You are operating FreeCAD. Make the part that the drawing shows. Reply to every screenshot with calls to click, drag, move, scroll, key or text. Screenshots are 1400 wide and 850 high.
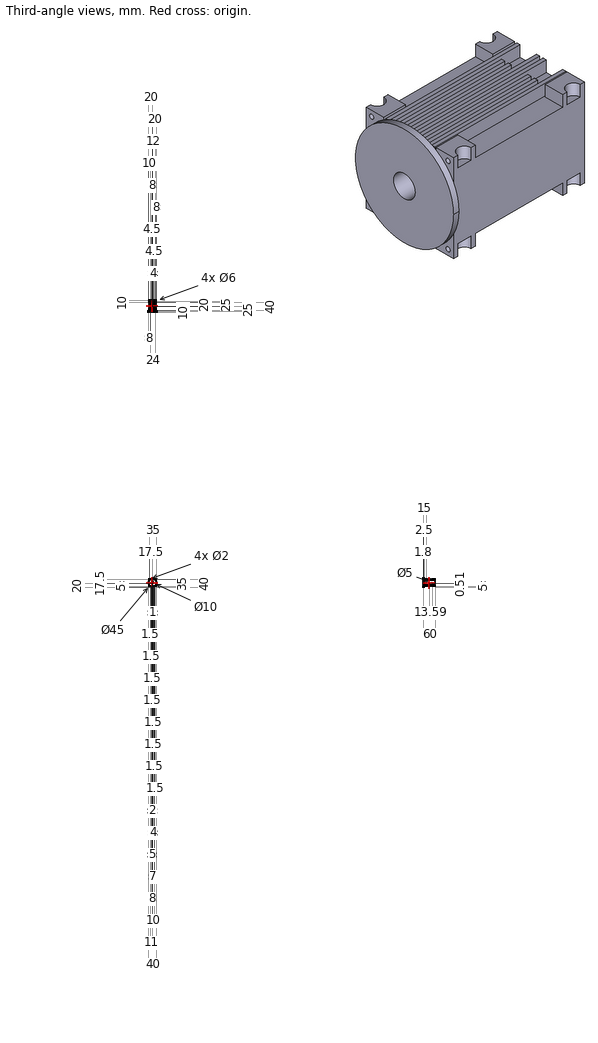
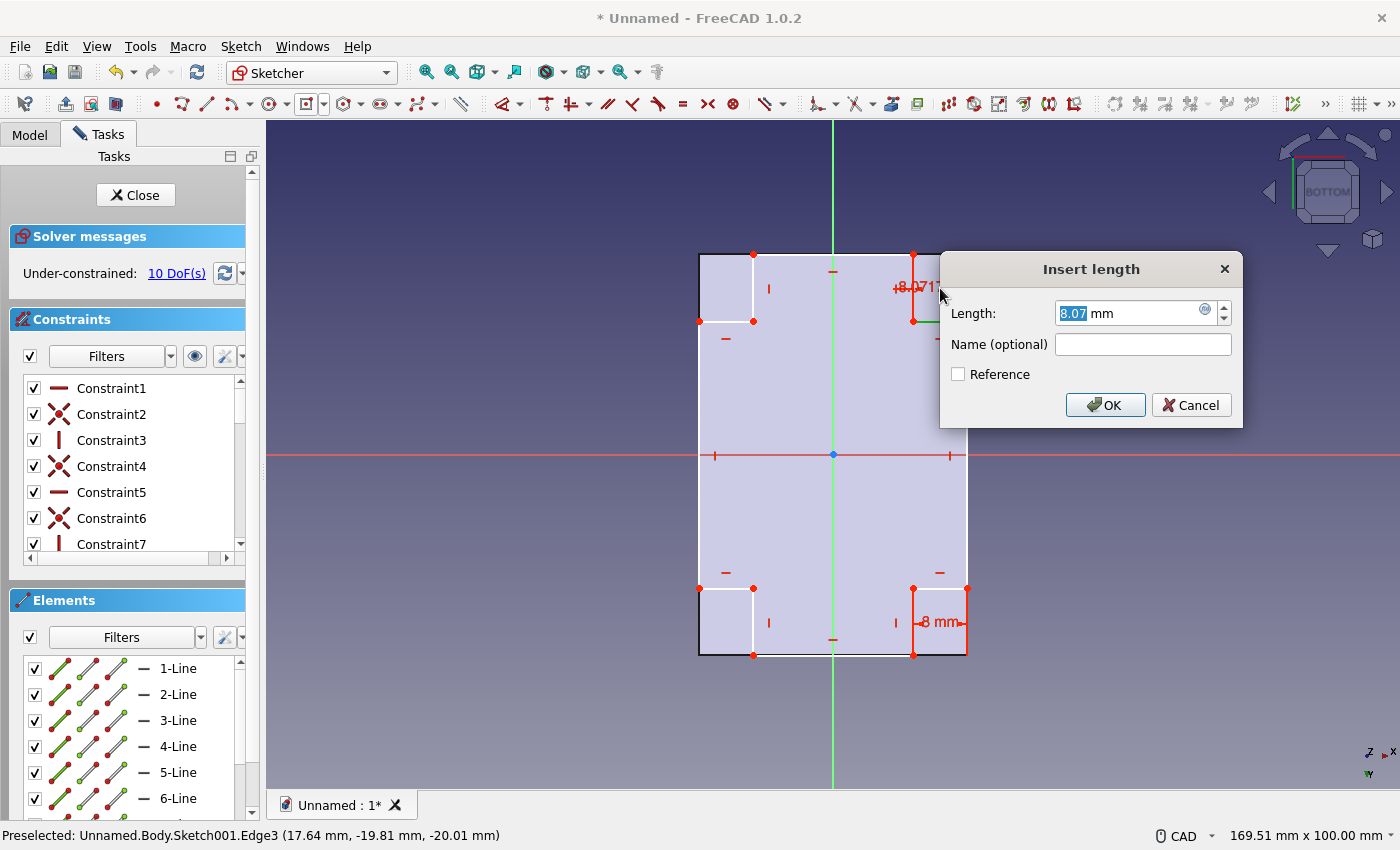
text(8)
key(Return)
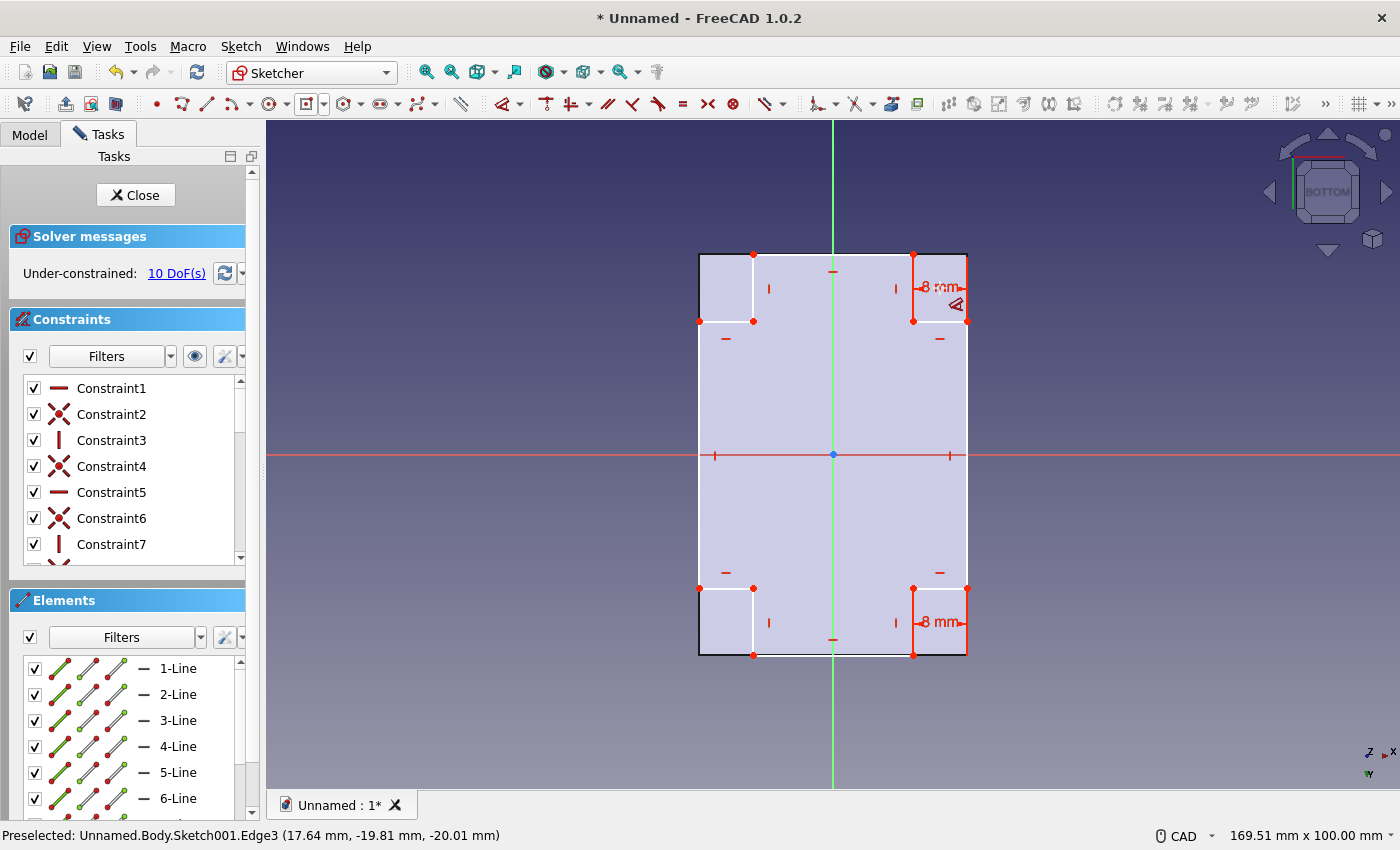
click(737, 322)
click(726, 288)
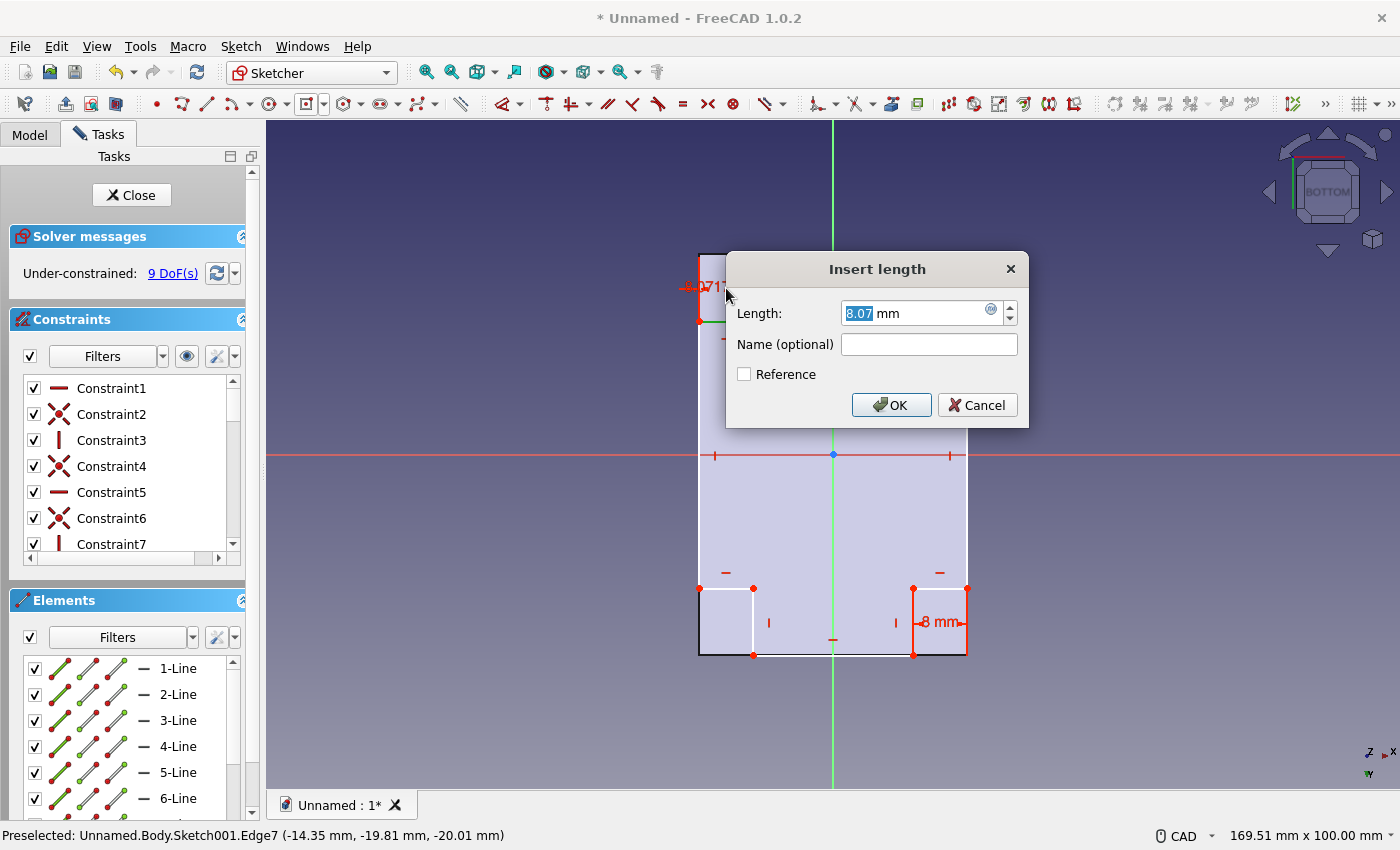
text(8)
key(Return)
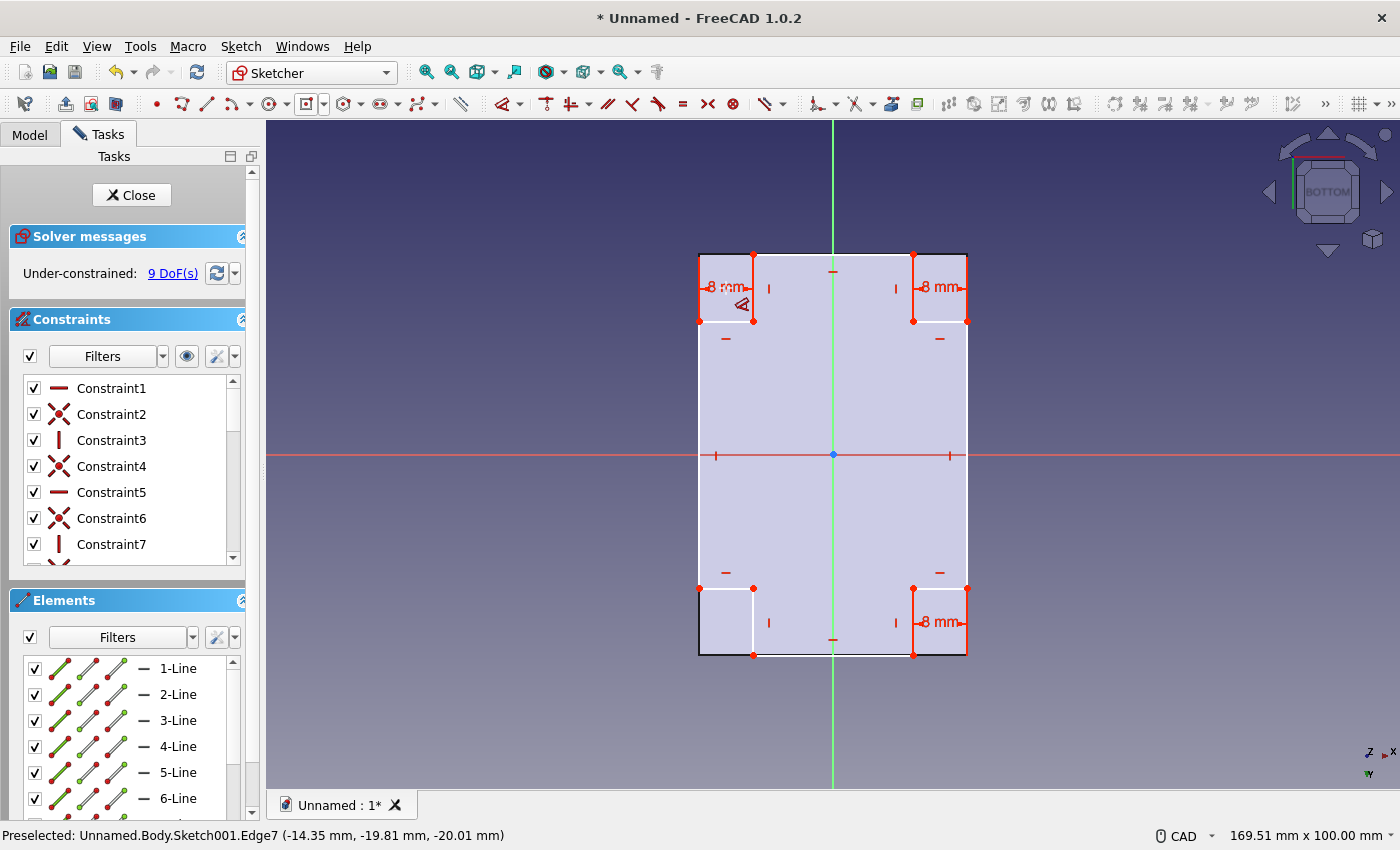
click(716, 589)
click(726, 623)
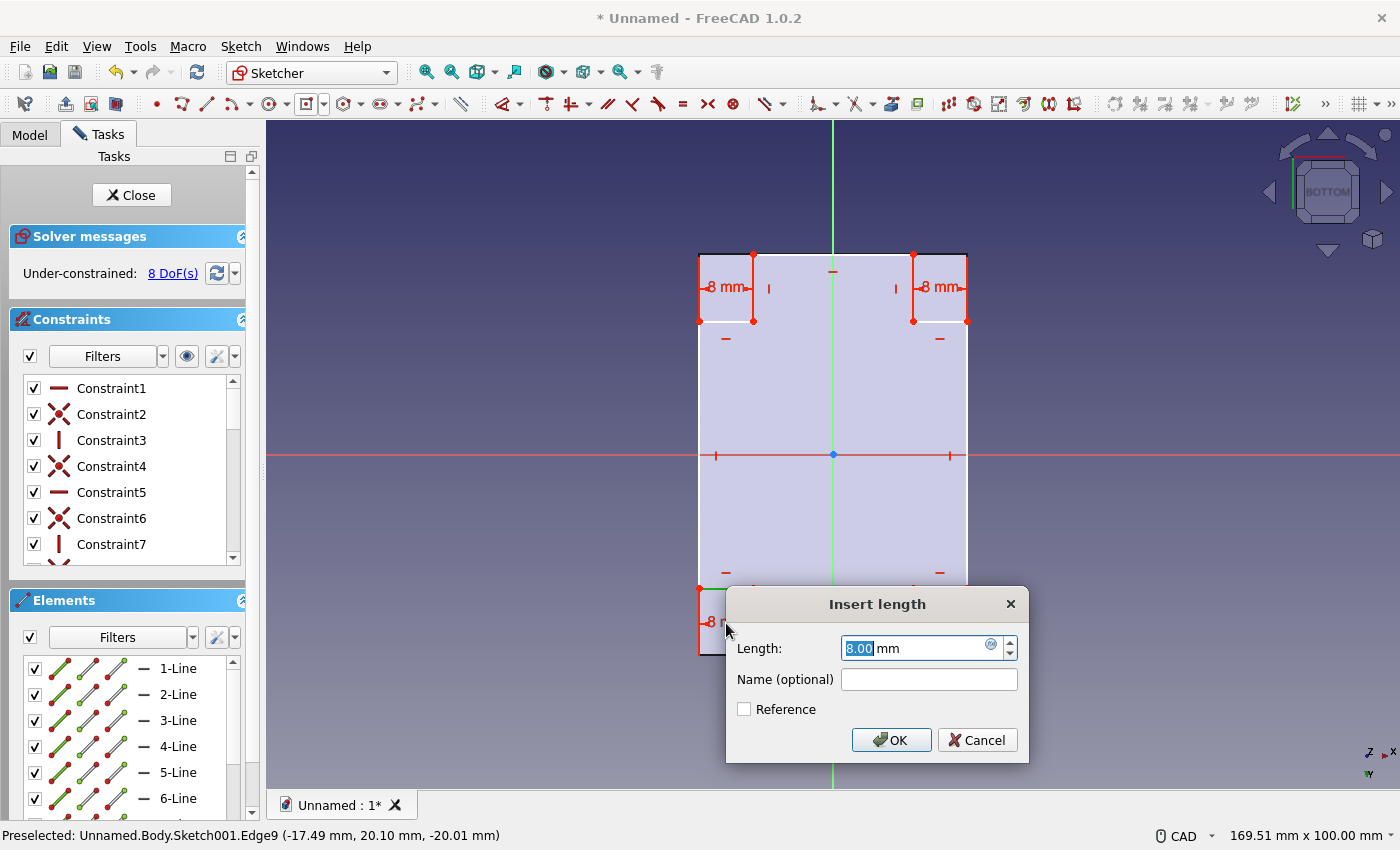
text(8)
key(Return)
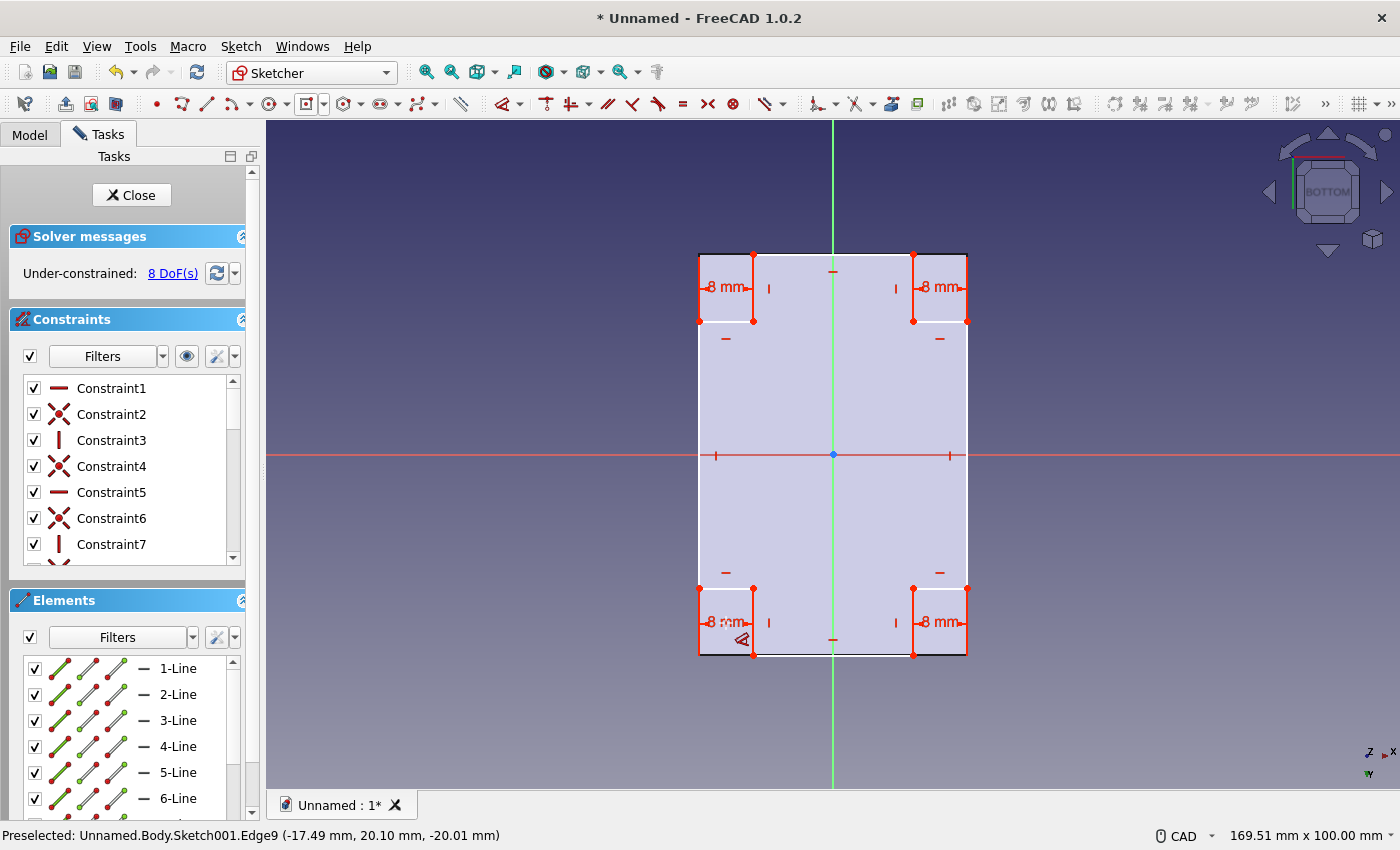
click(967, 509)
click(1001, 394)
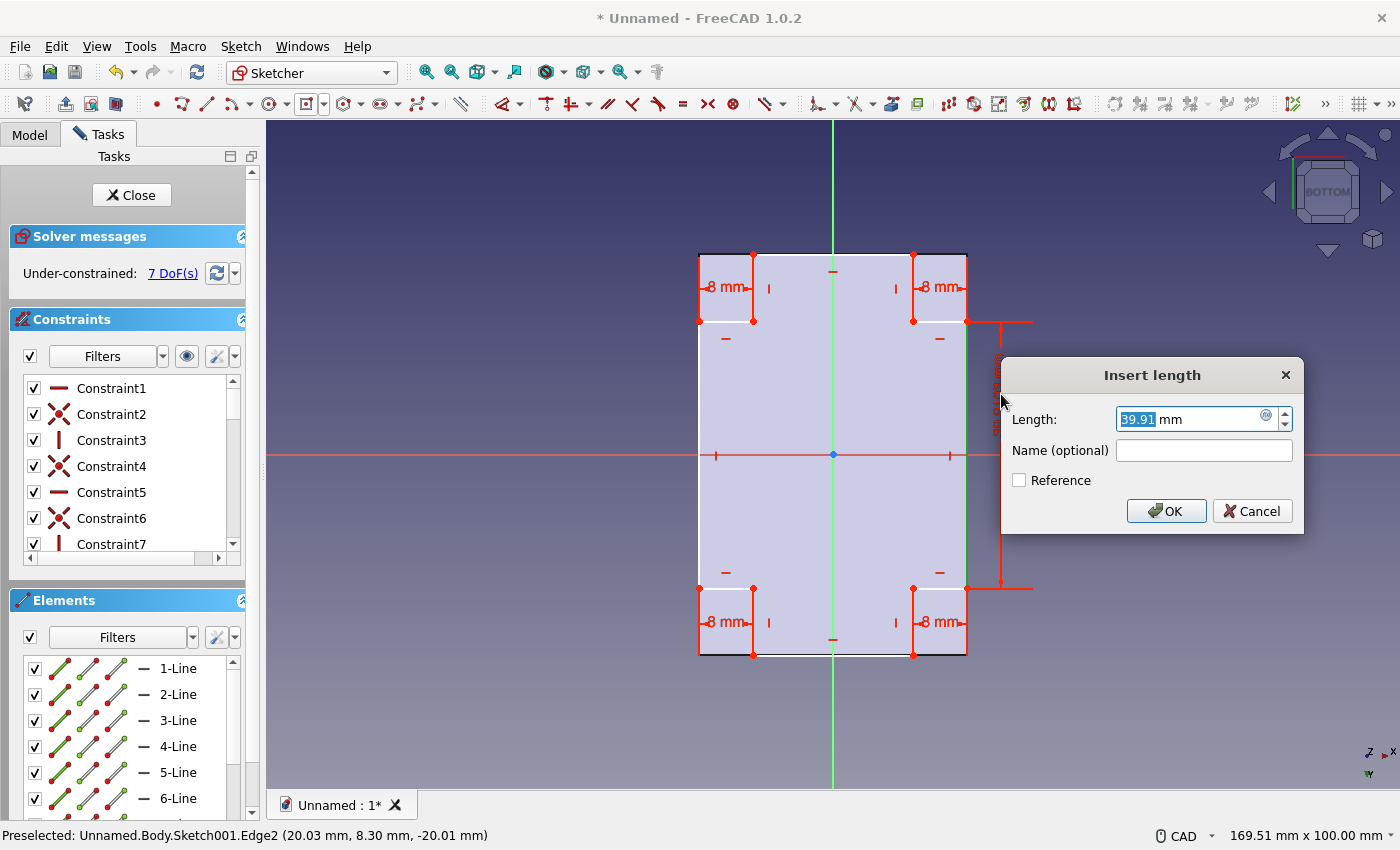
text(40)
key(Return)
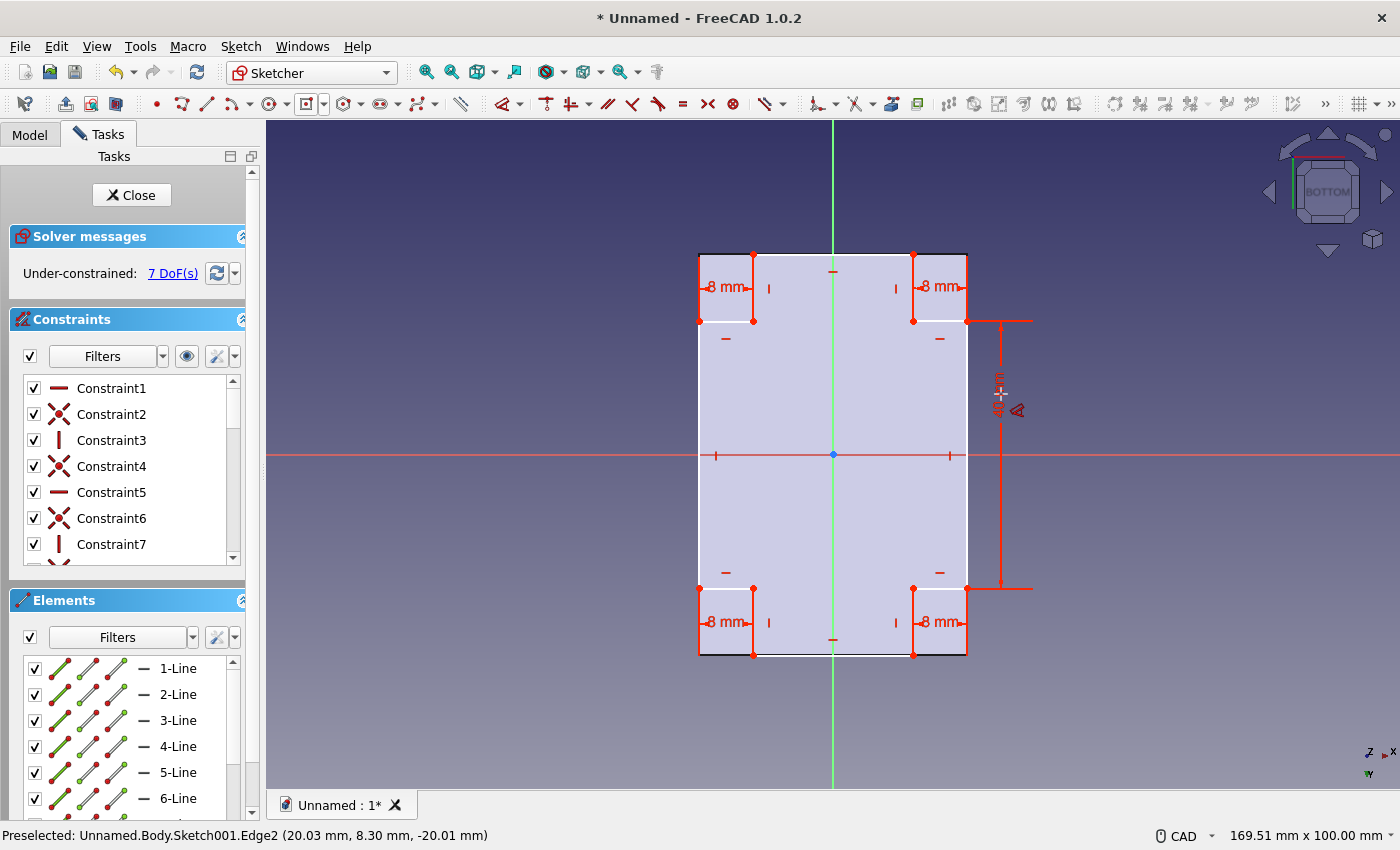
click(913, 301)
click(947, 265)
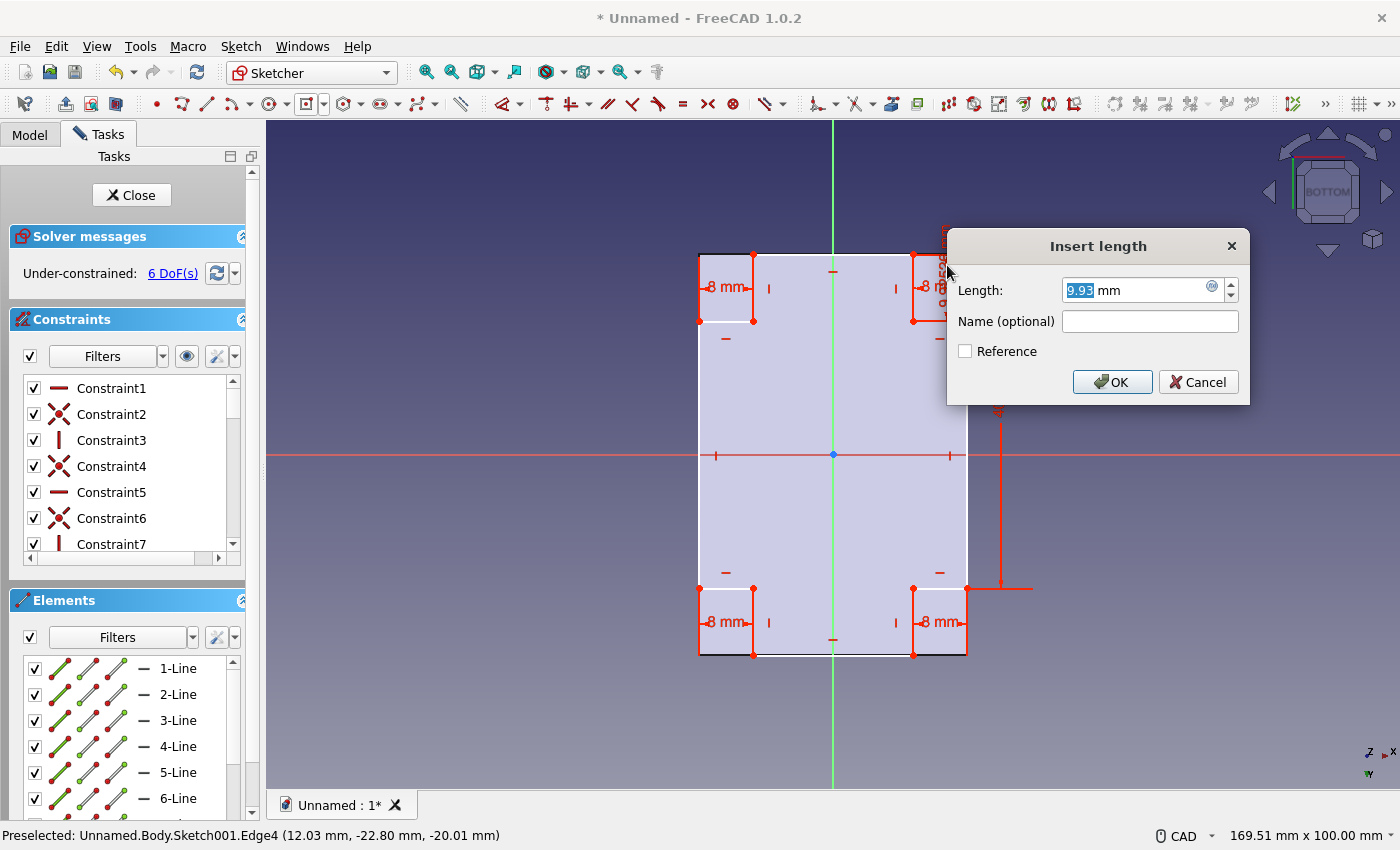
text(10)
key(Return)